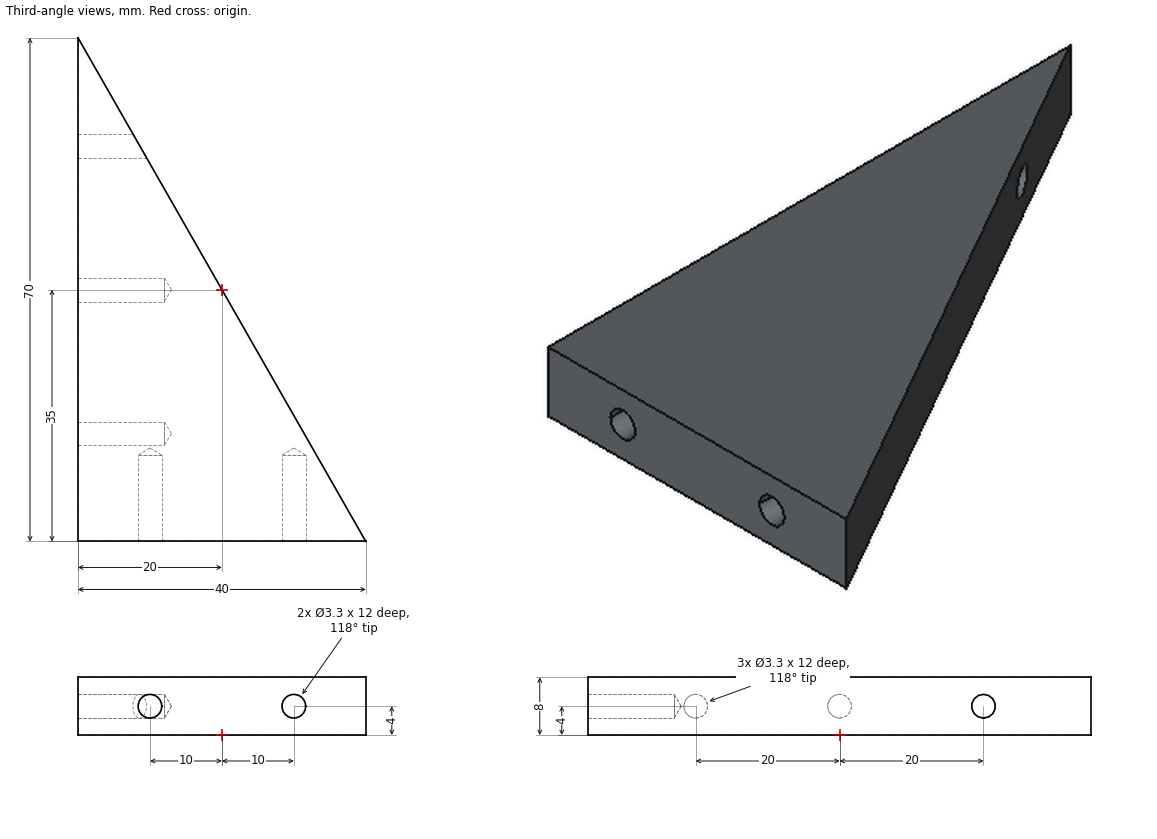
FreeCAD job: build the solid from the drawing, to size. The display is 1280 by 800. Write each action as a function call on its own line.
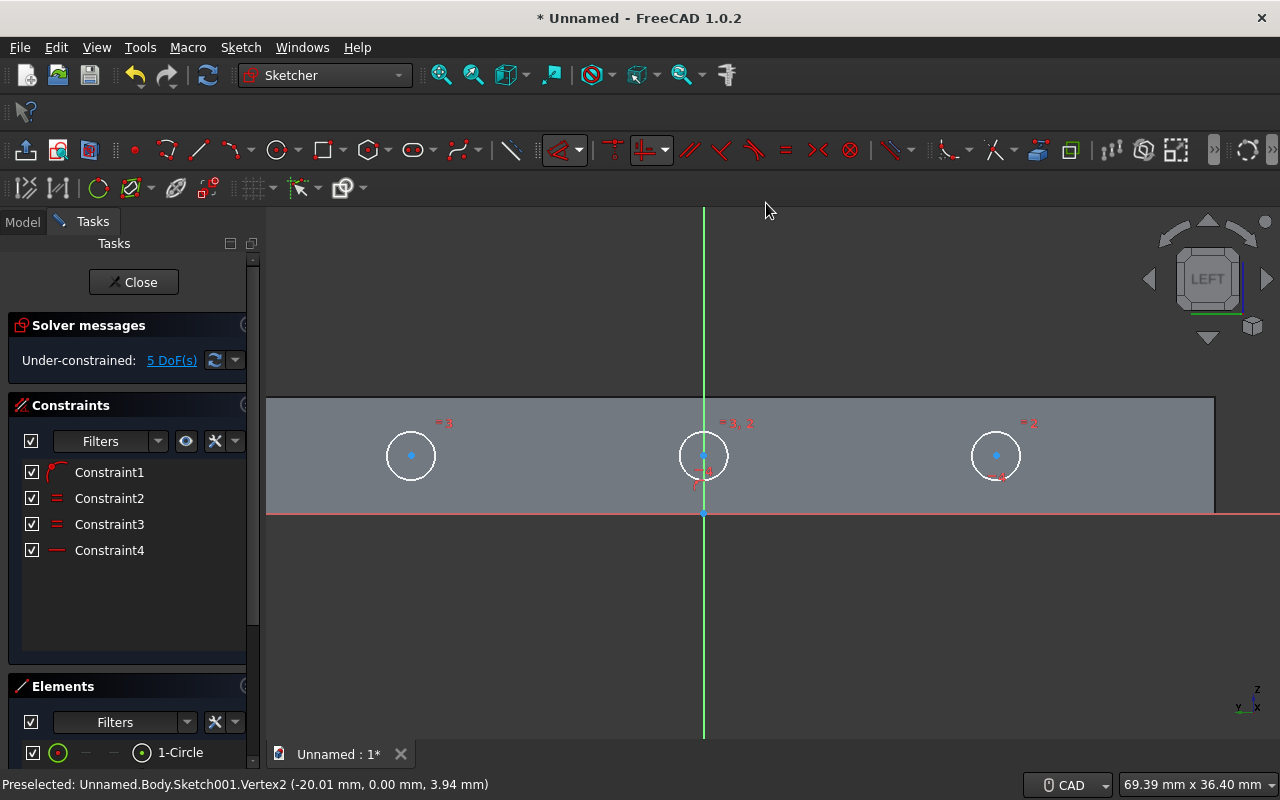
click(704, 456)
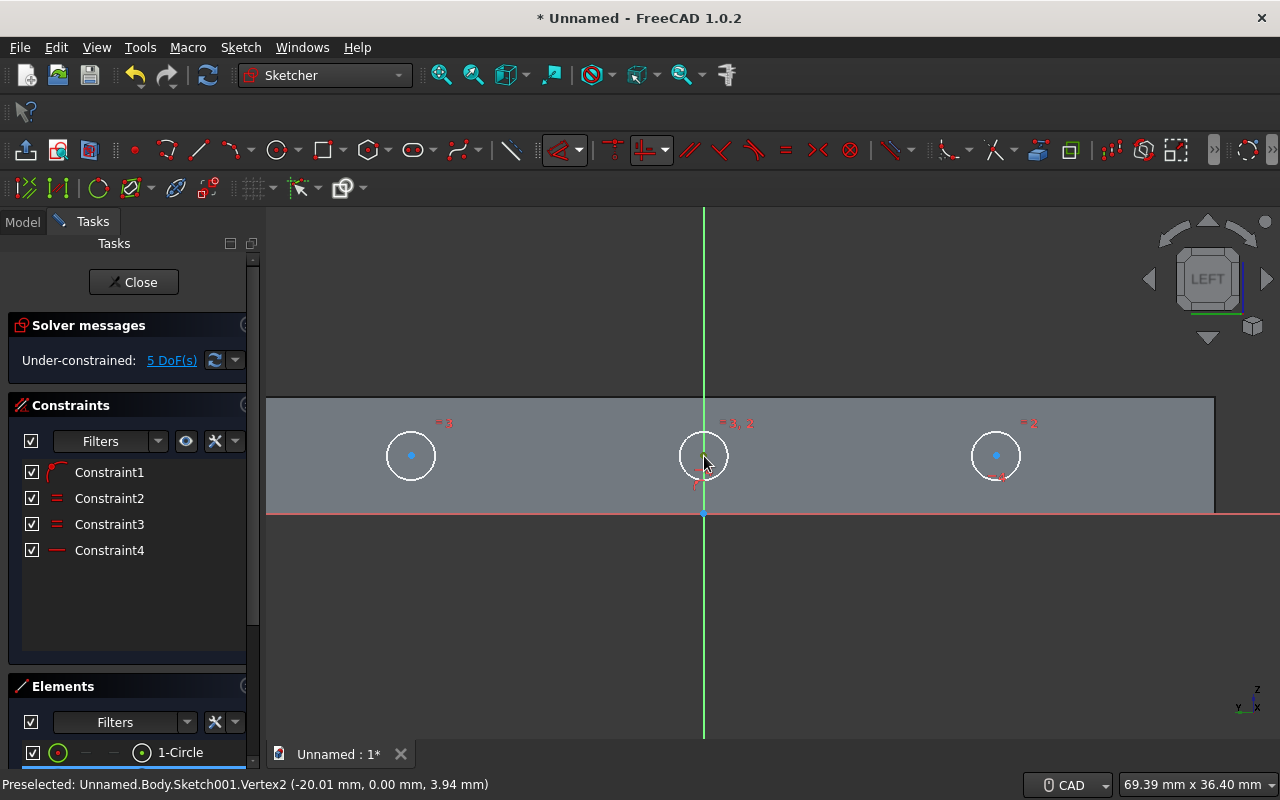
click(411, 456)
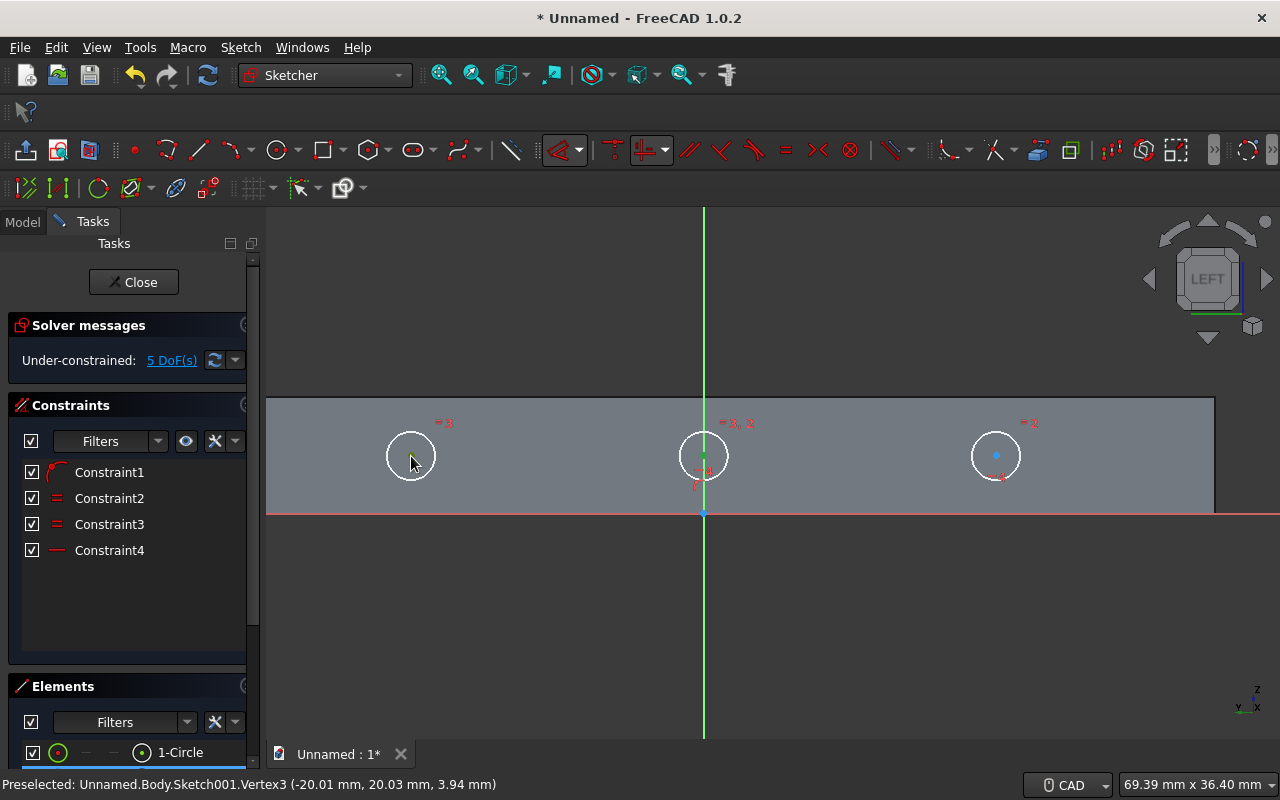
key(h)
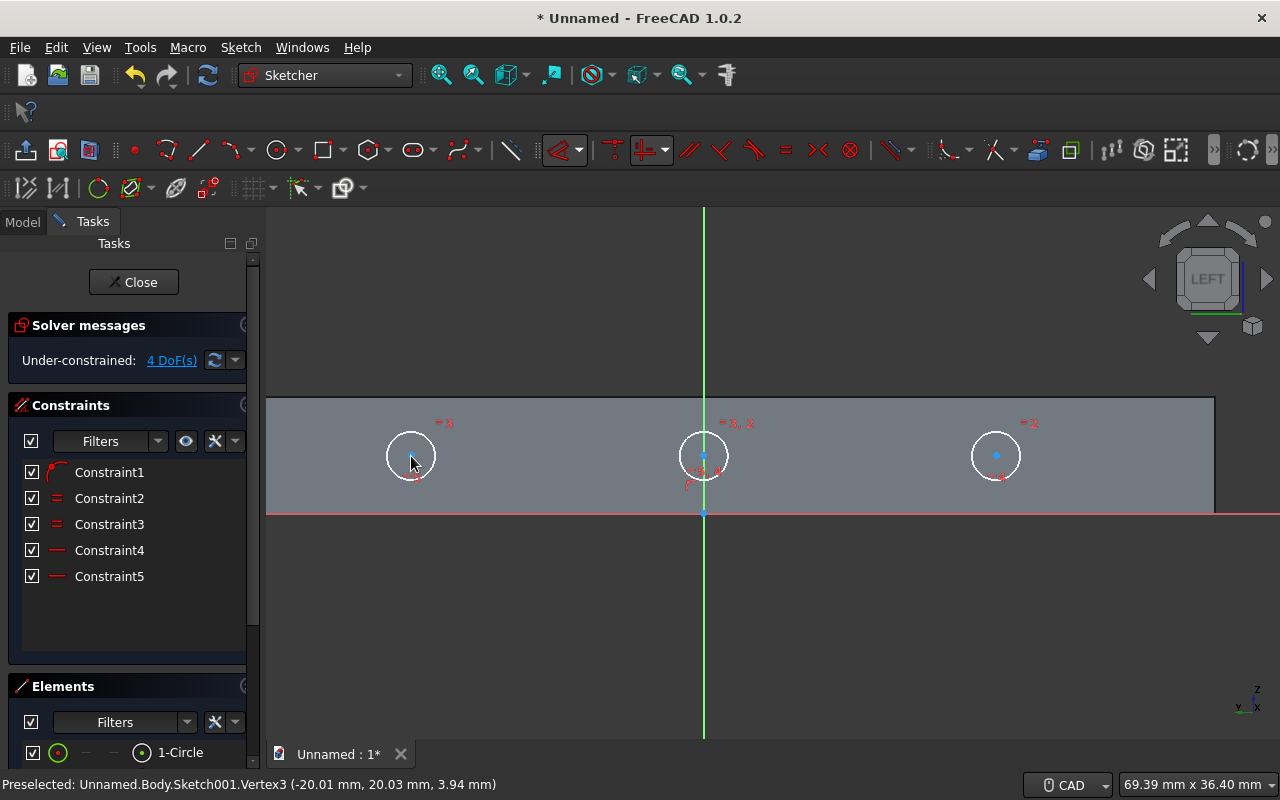
click(1013, 439)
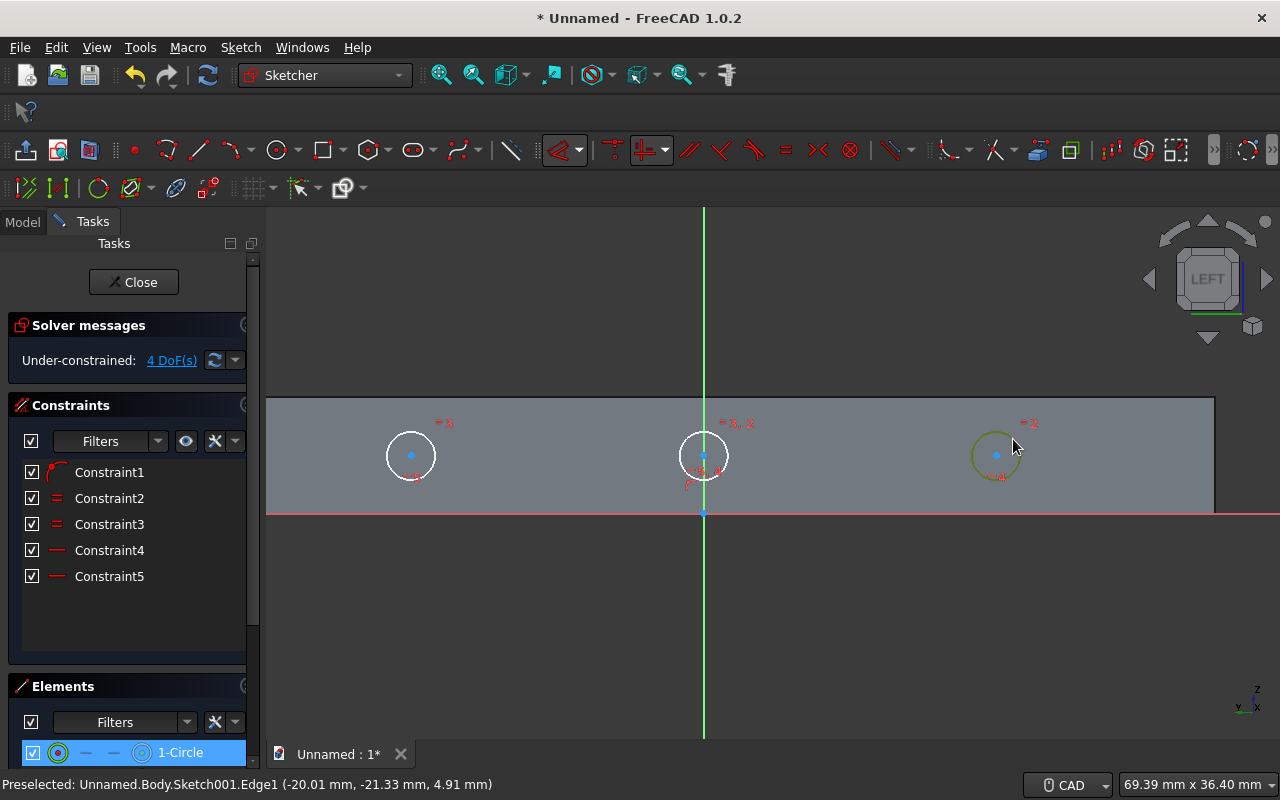
click(582, 150)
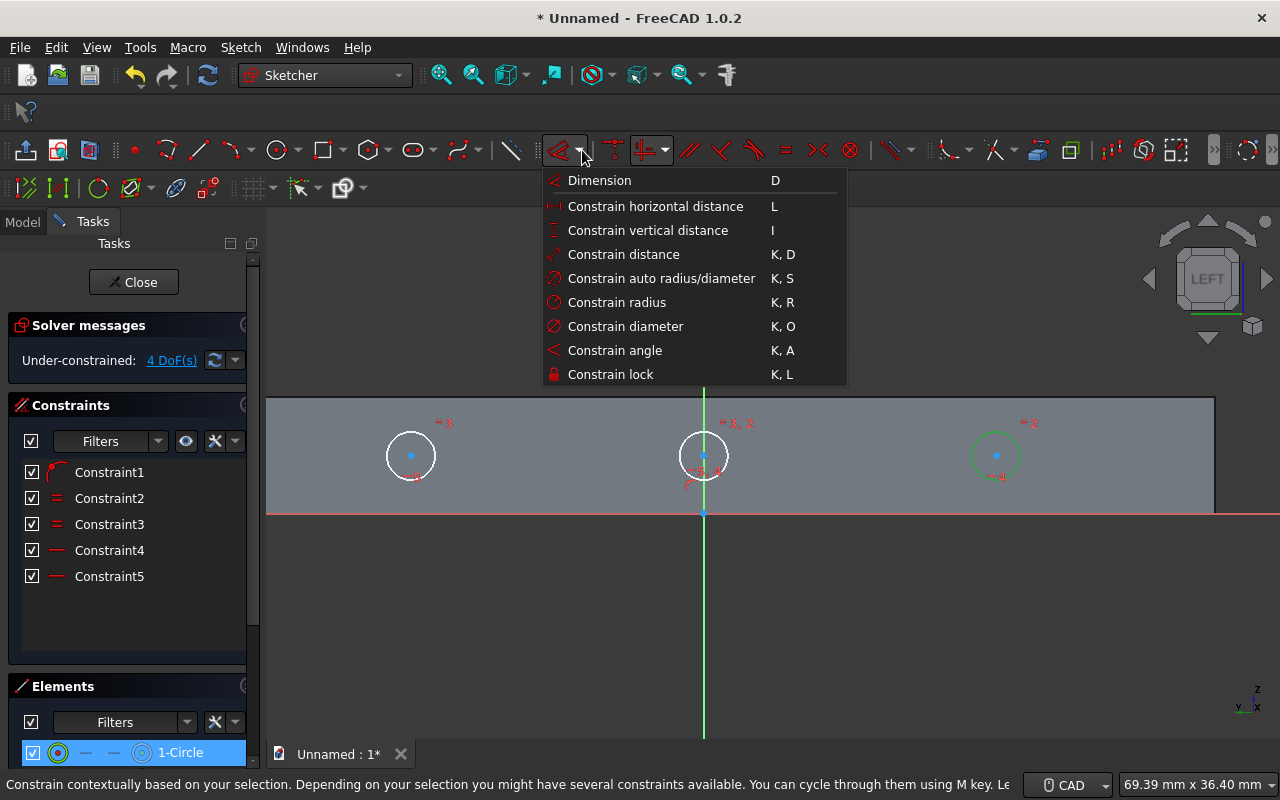
click(695, 326)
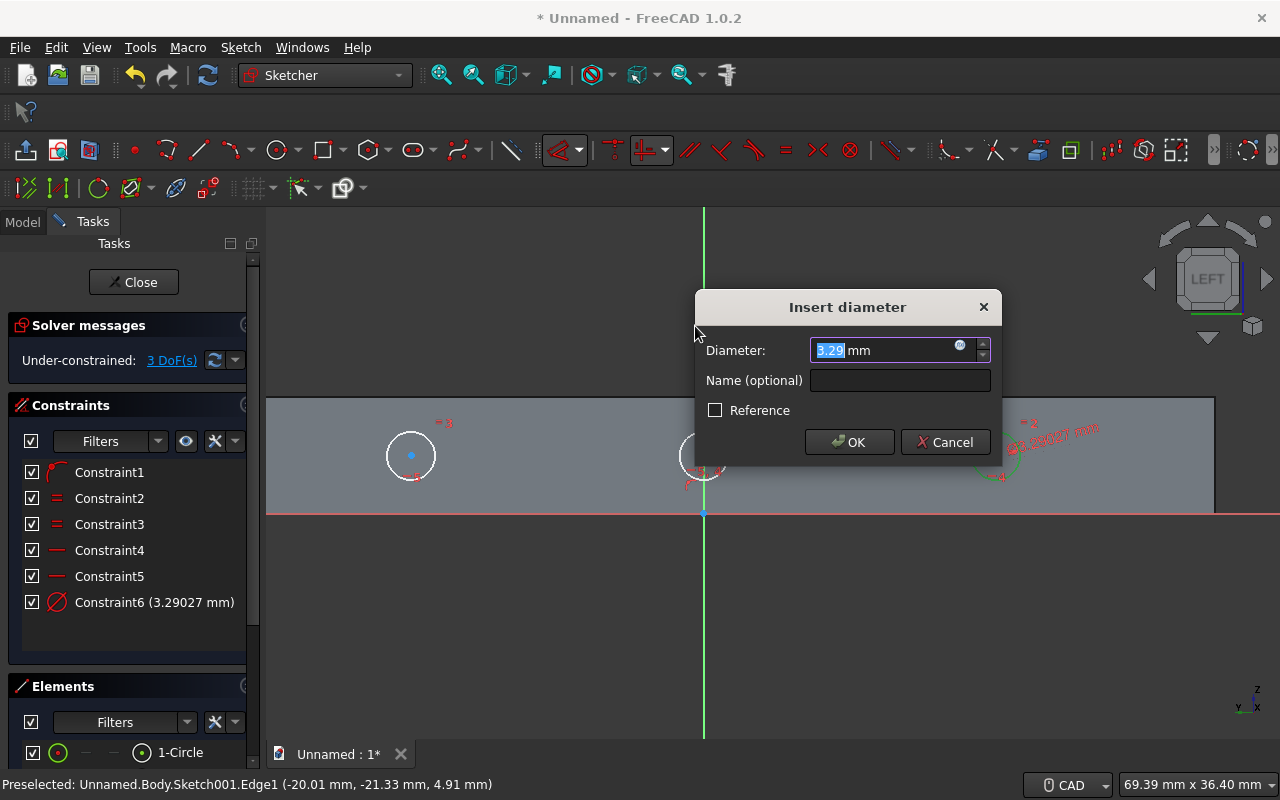
text(3.3)
key(Return)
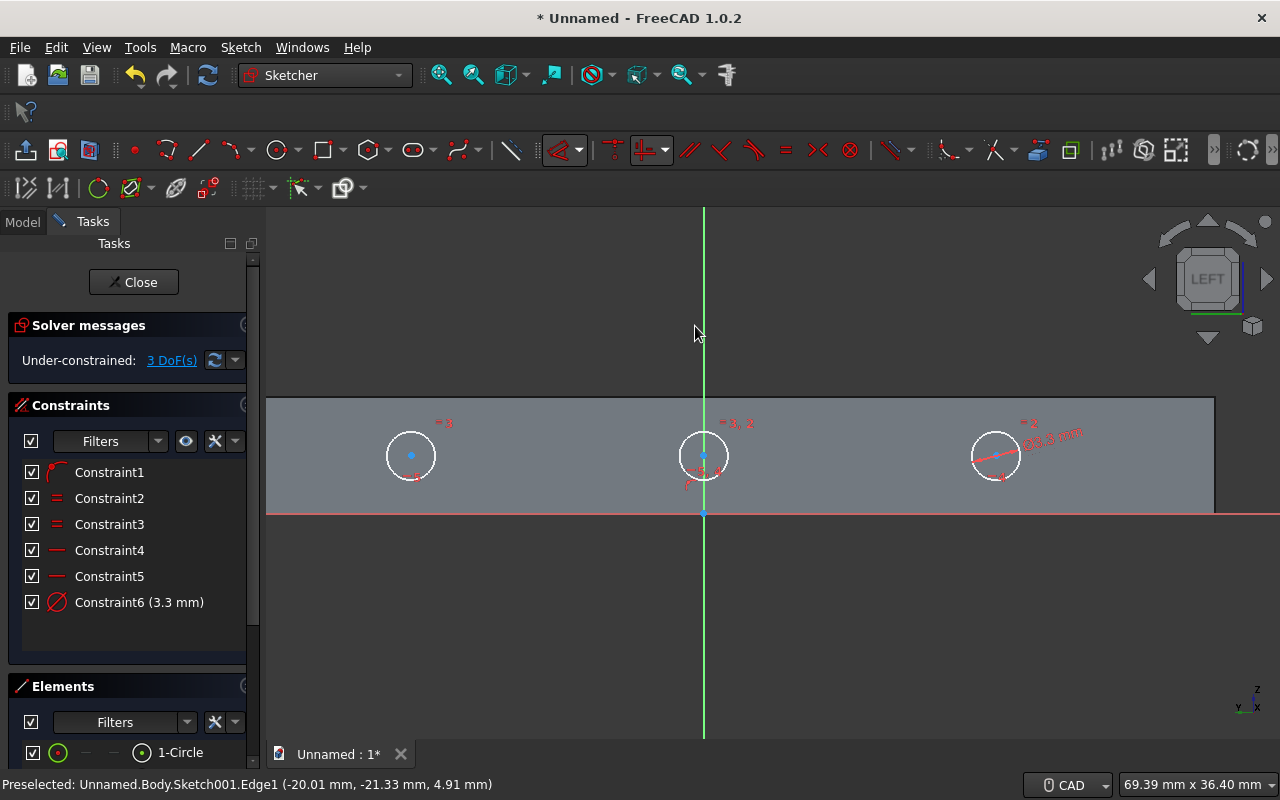
click(996, 456)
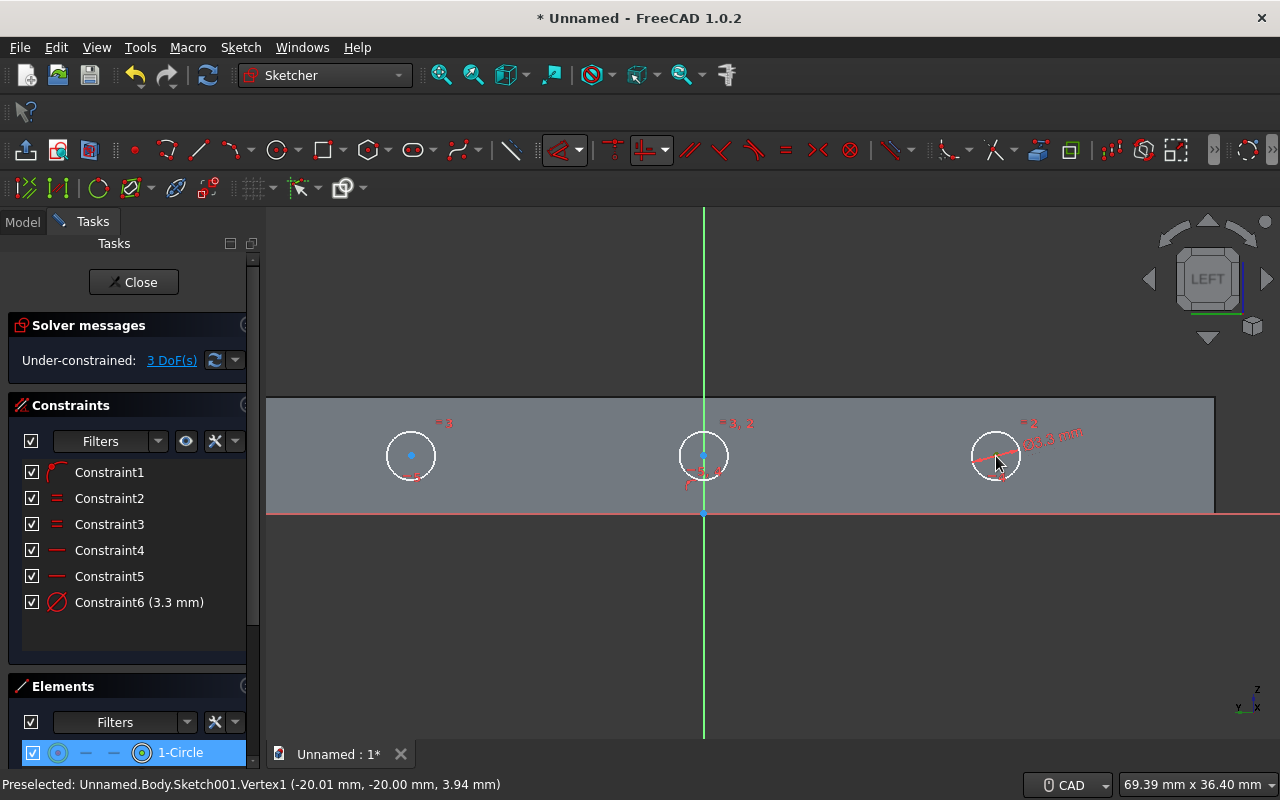
key(i)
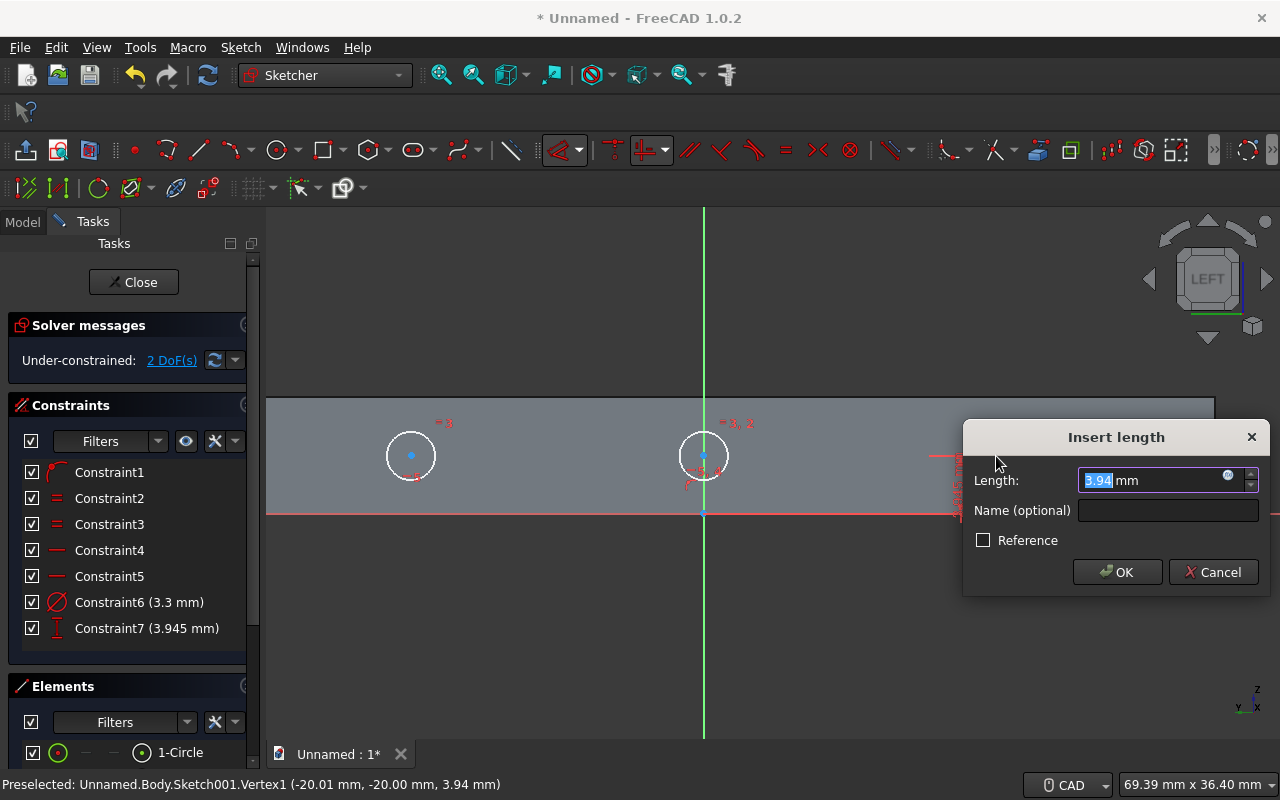
text(4)
key(Return)